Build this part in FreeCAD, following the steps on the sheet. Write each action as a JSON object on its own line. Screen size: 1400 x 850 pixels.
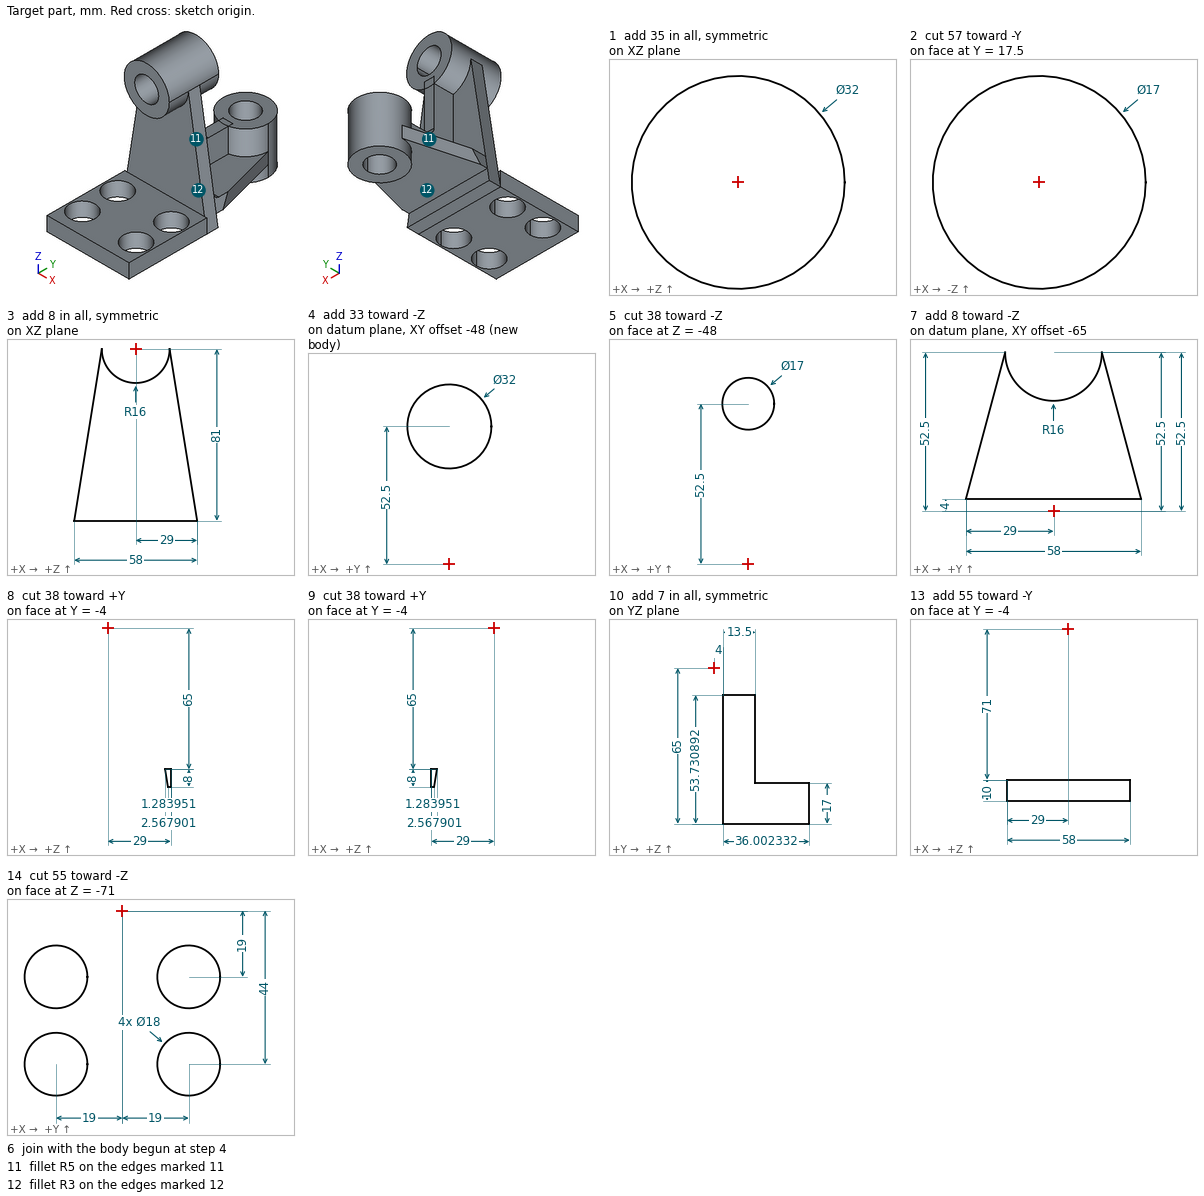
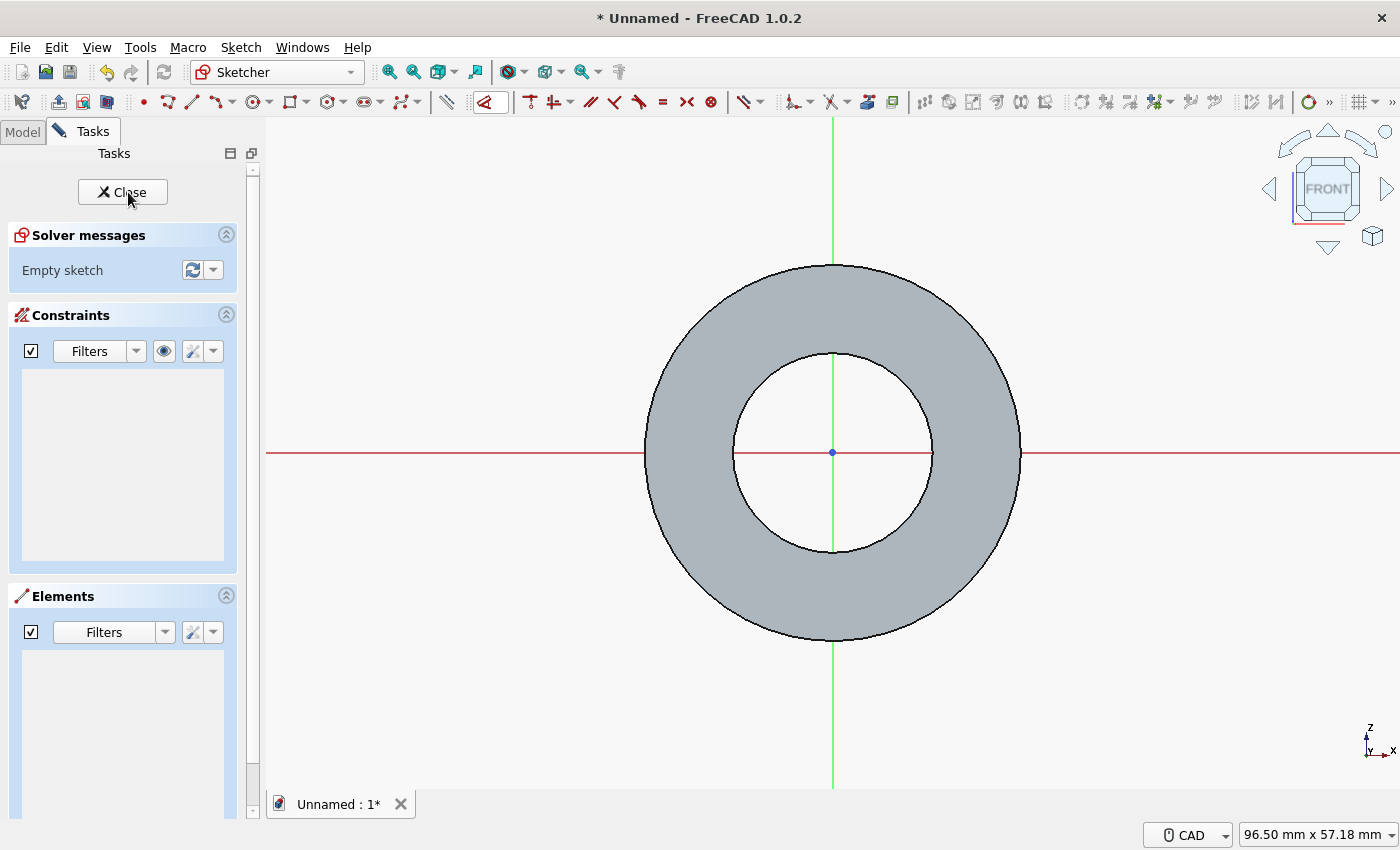
{"action": "key", "text": "q s"}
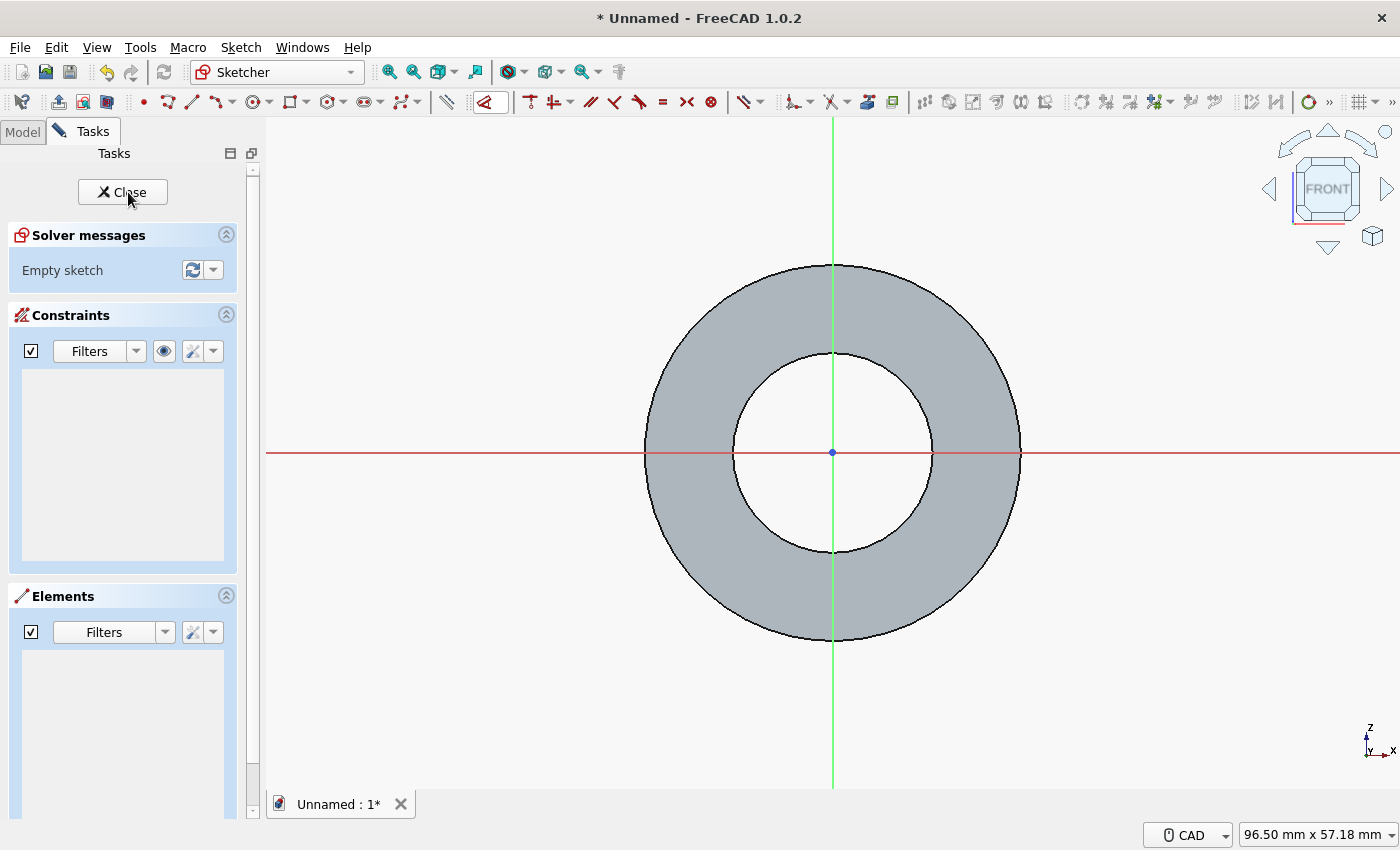
{"action": "scroll", "coordinate": [709, 145], "scroll_direction": "down", "scroll_amount": 4}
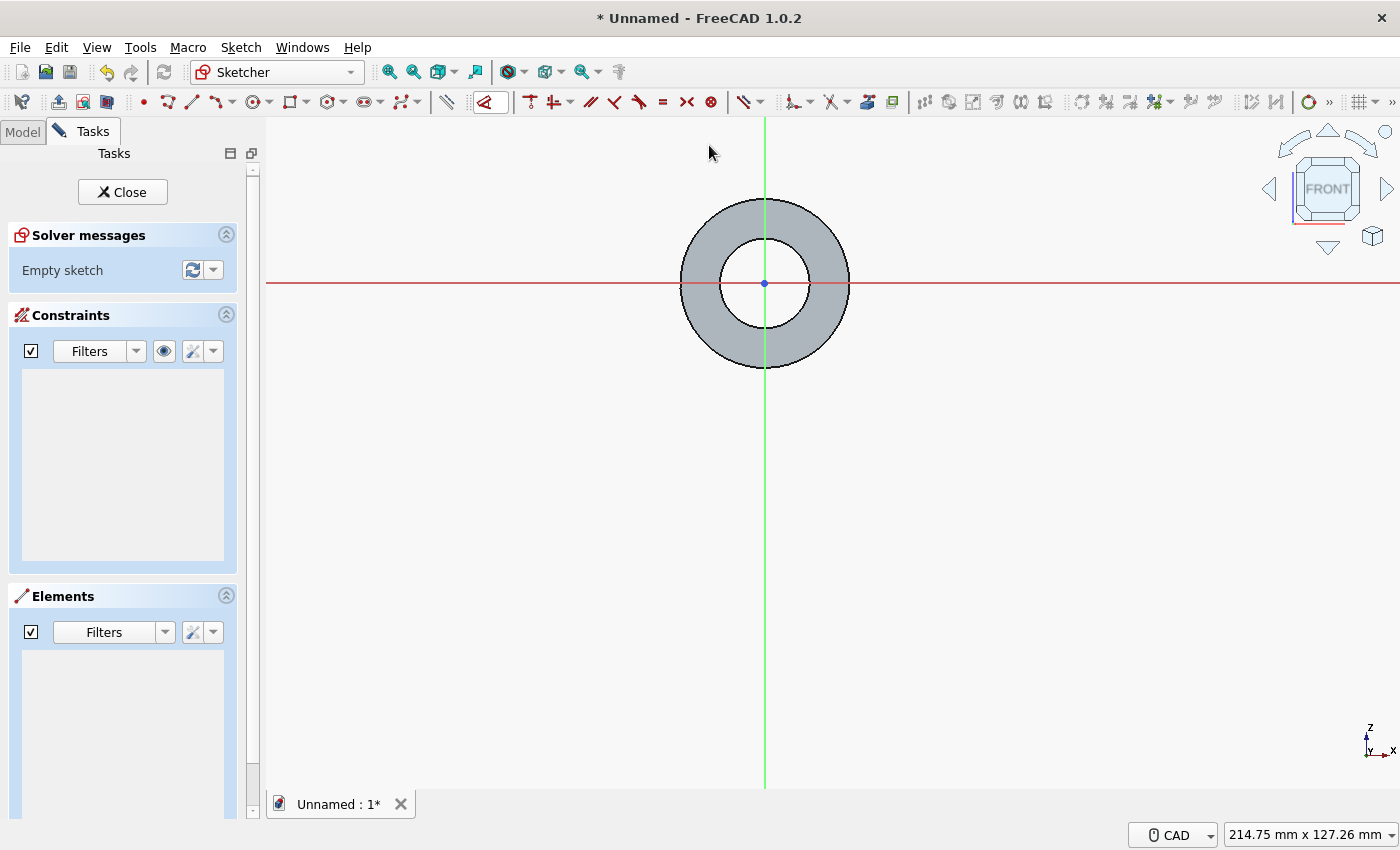
{"action": "key", "text": "g m"}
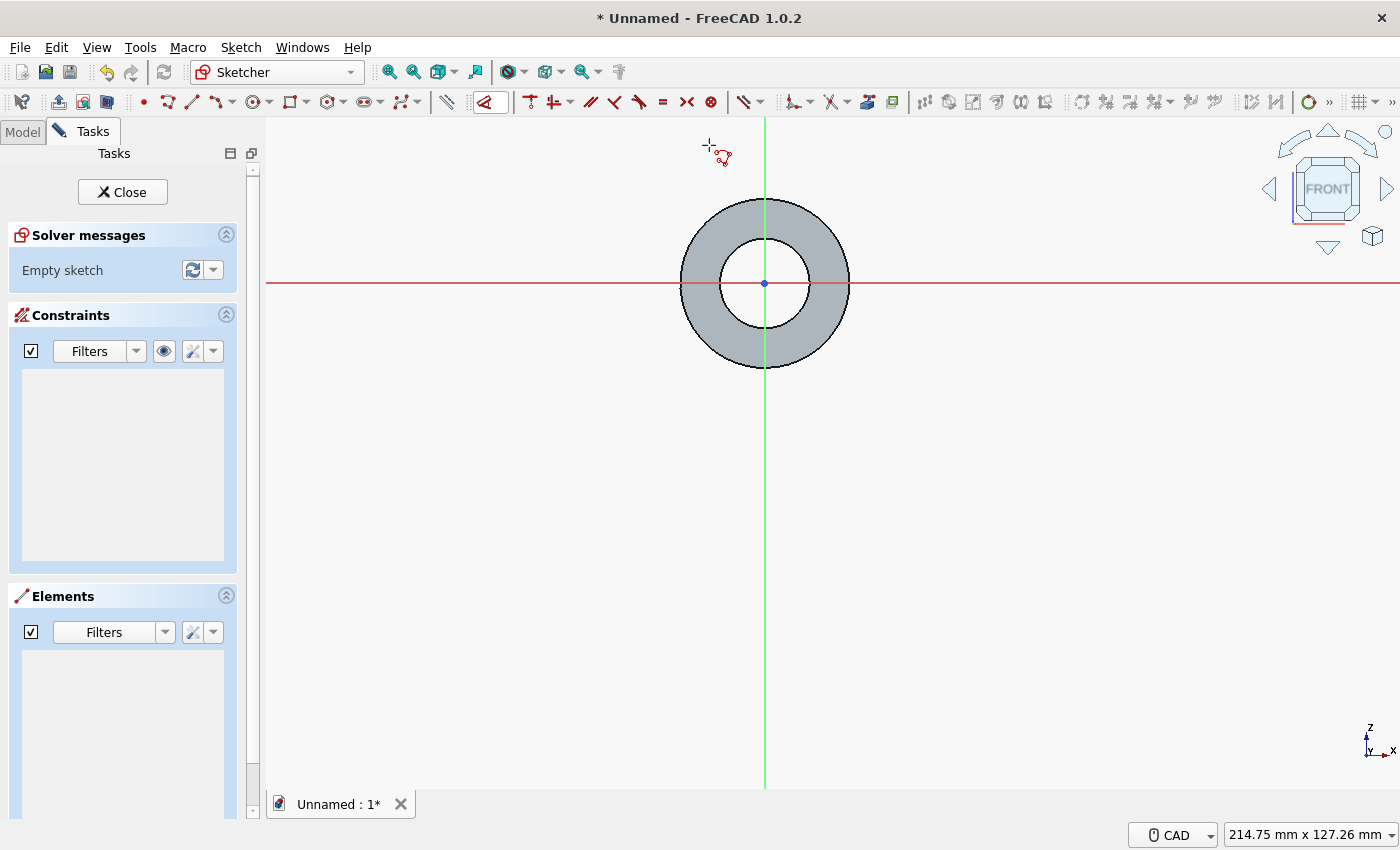
{"action": "left_click", "coordinate": [849, 283]}
{"action": "left_click", "coordinate": [918, 711]}
{"action": "left_click", "coordinate": [612, 711]}
{"action": "left_click", "coordinate": [680, 283]}
{"action": "right_click", "coordinate": [680, 283]}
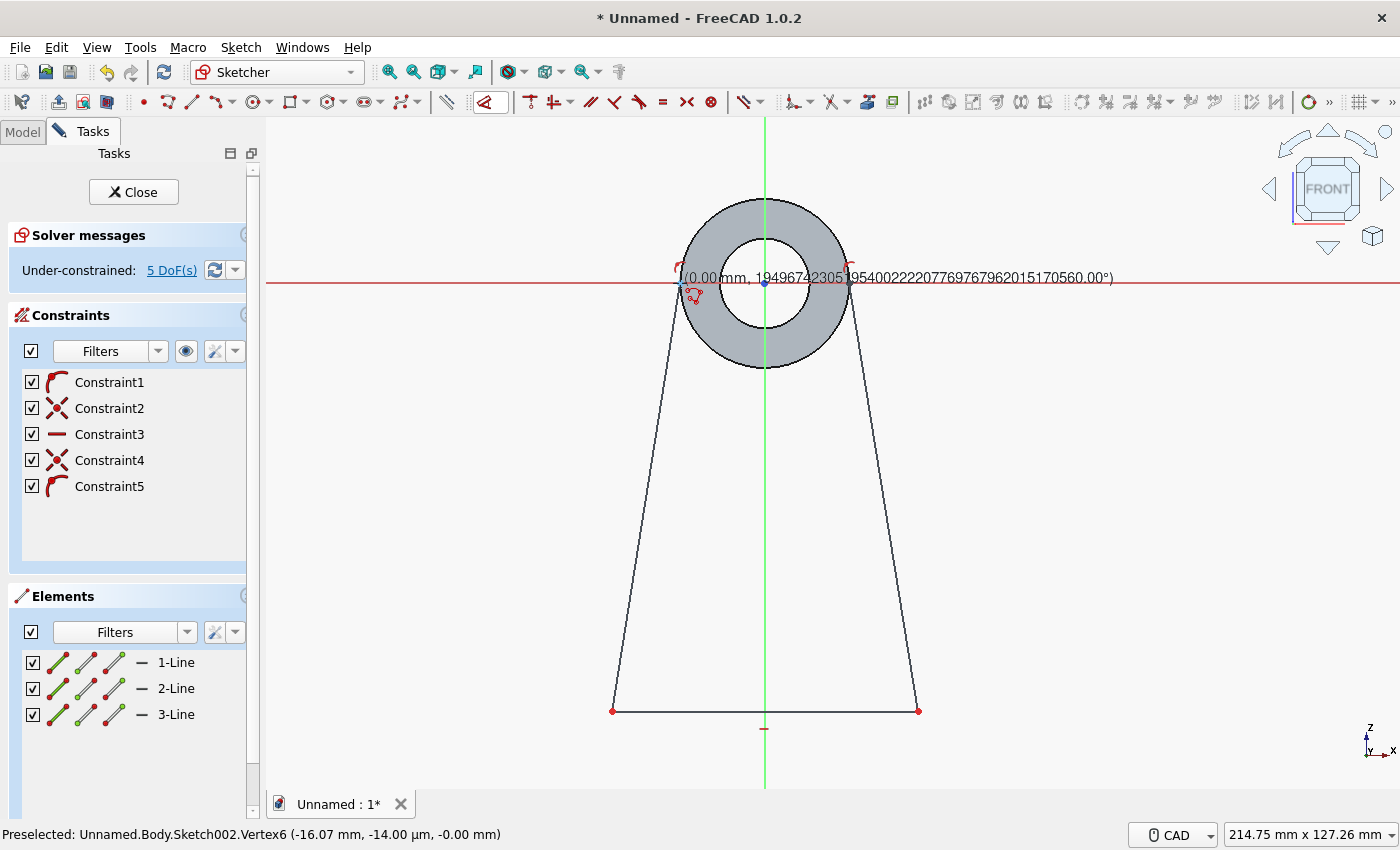
{"action": "key", "text": "g 3 a"}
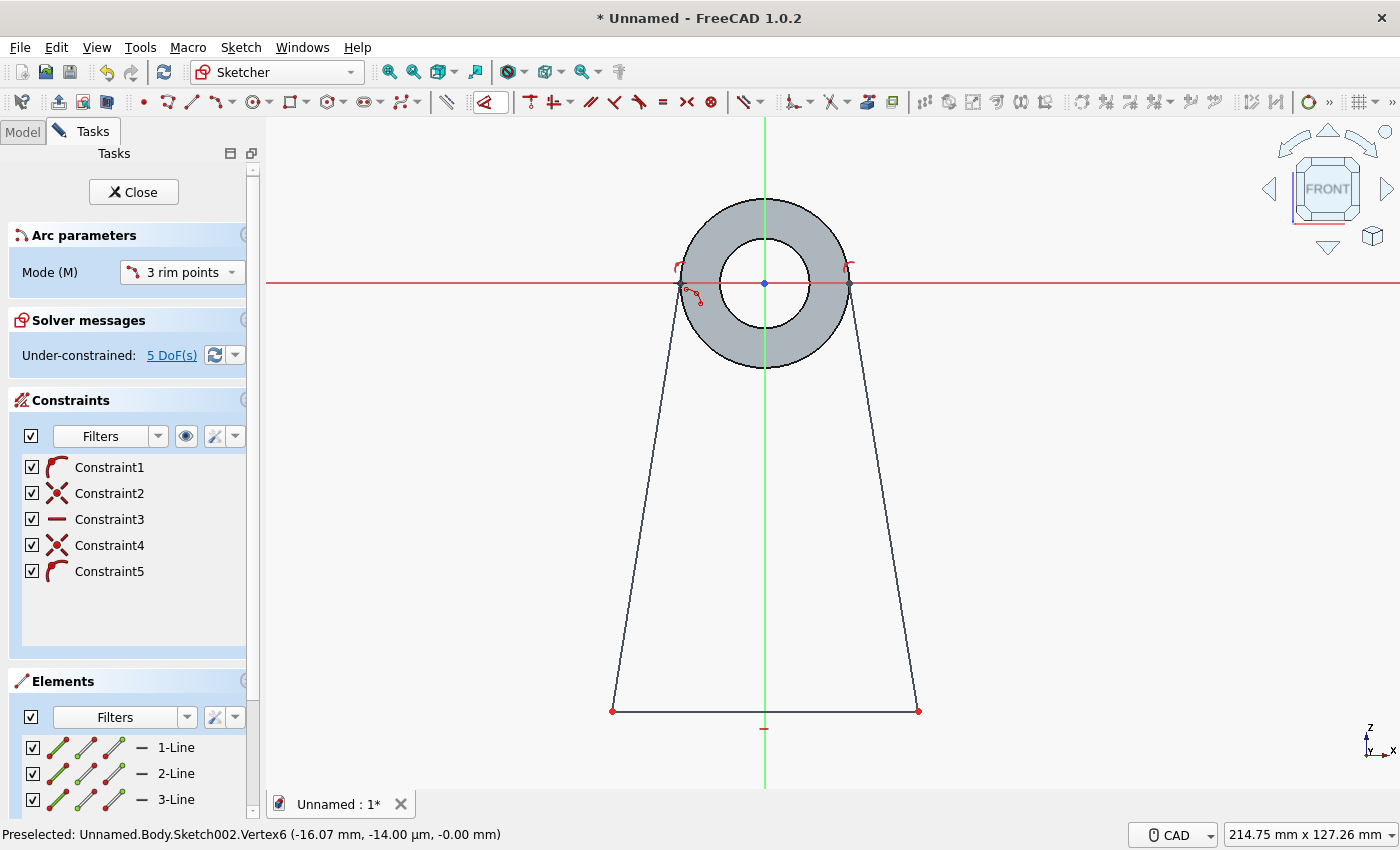
{"action": "left_click", "coordinate": [680, 283]}
{"action": "left_click", "coordinate": [849, 283]}
{"action": "left_click", "coordinate": [739, 364]}
{"action": "key", "text": "Escape"}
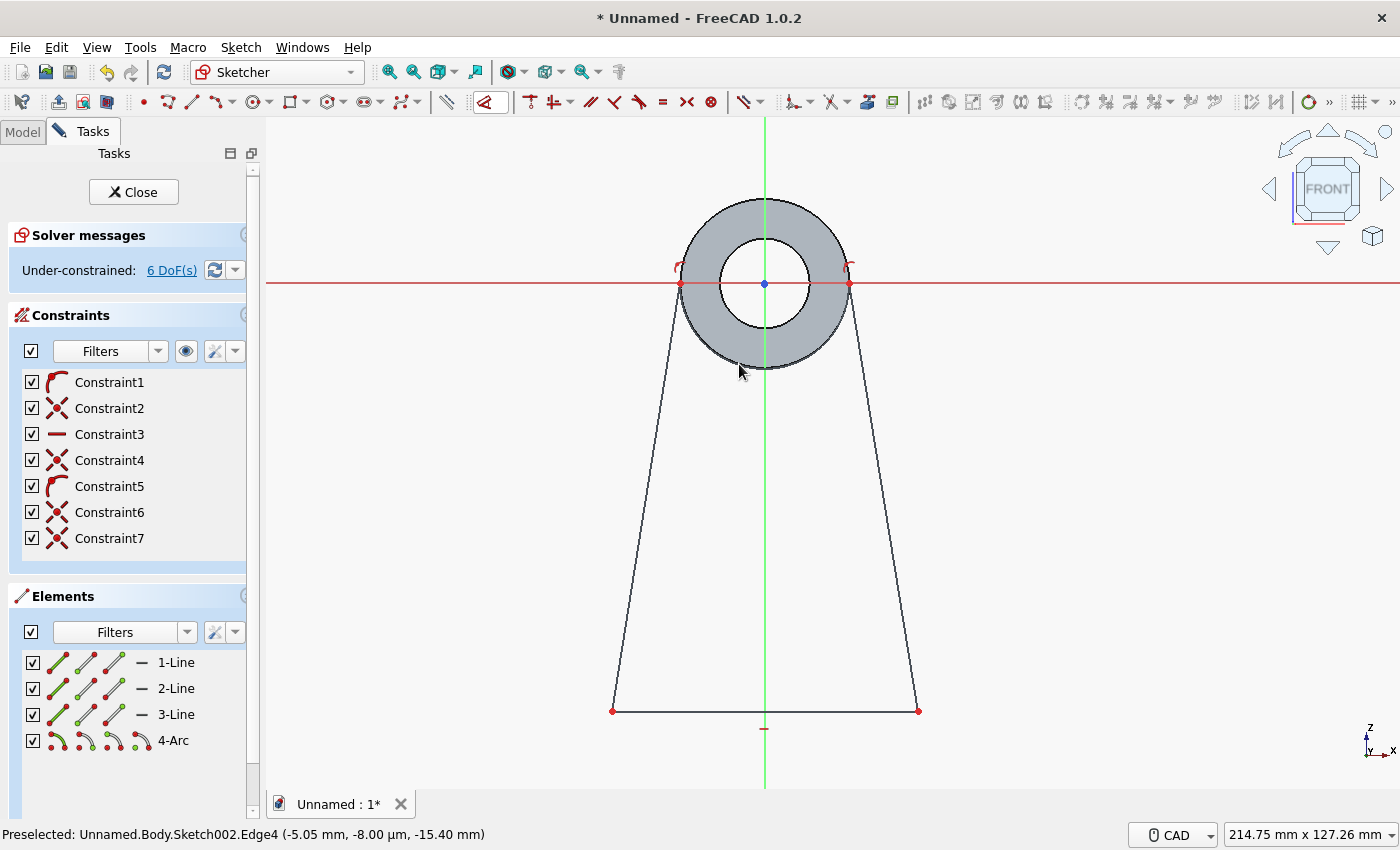
{"action": "left_click_drag", "start_coordinate": [755, 273], "coordinate": [775, 294]}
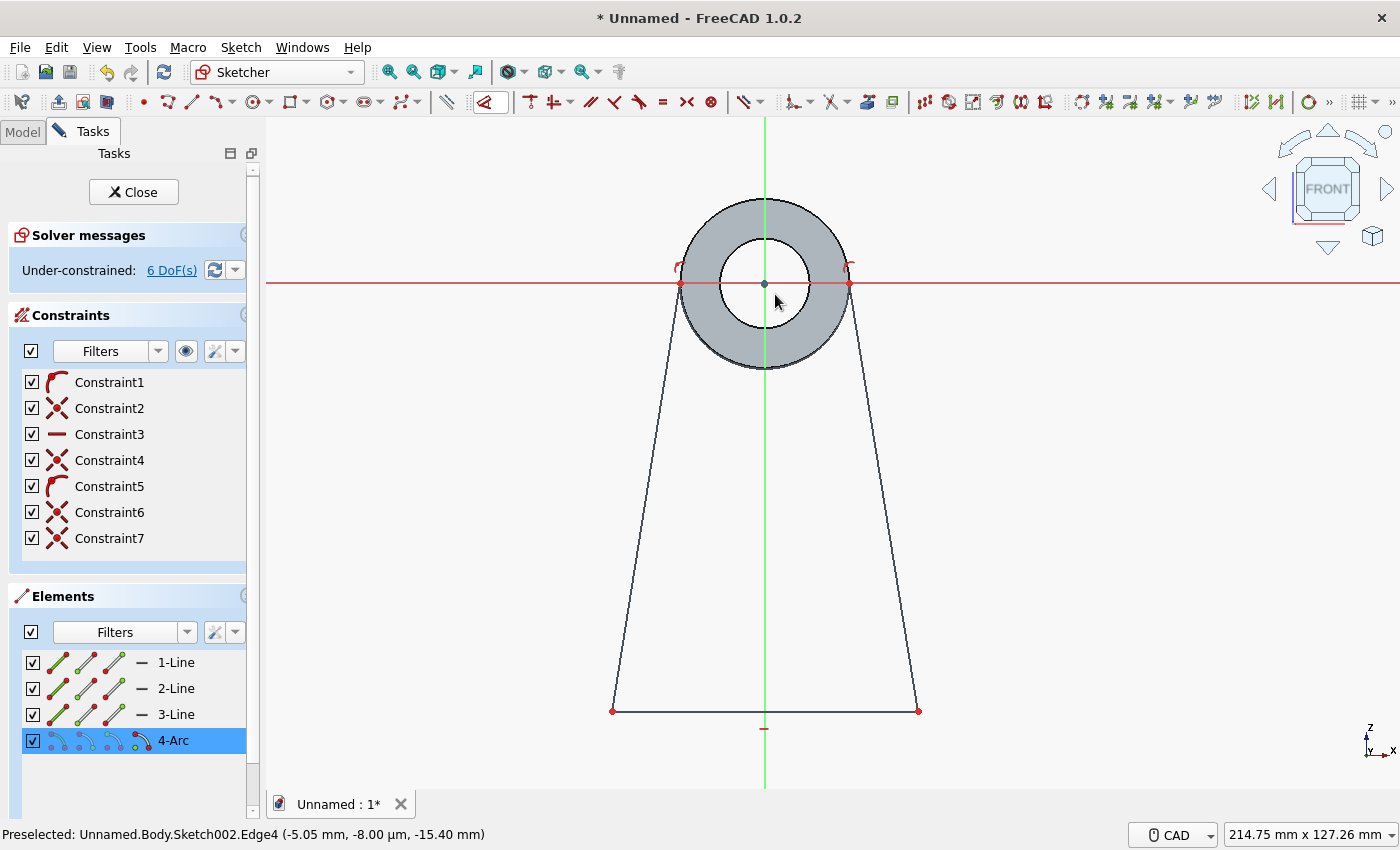
{"action": "left_click", "coordinate": [530, 102]}